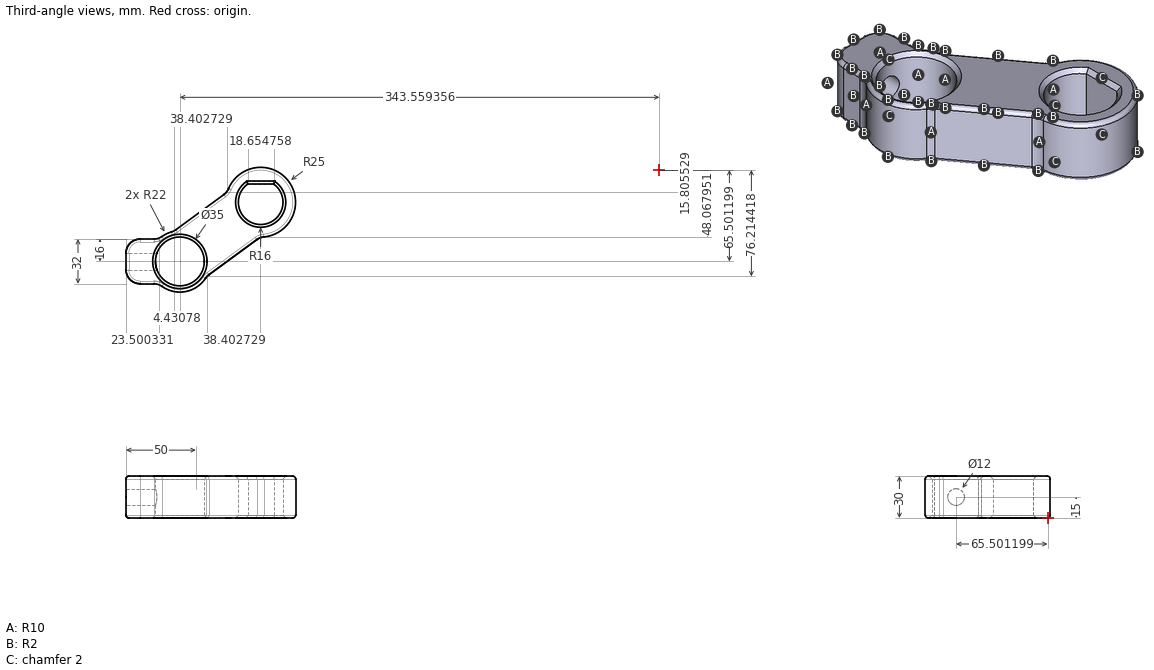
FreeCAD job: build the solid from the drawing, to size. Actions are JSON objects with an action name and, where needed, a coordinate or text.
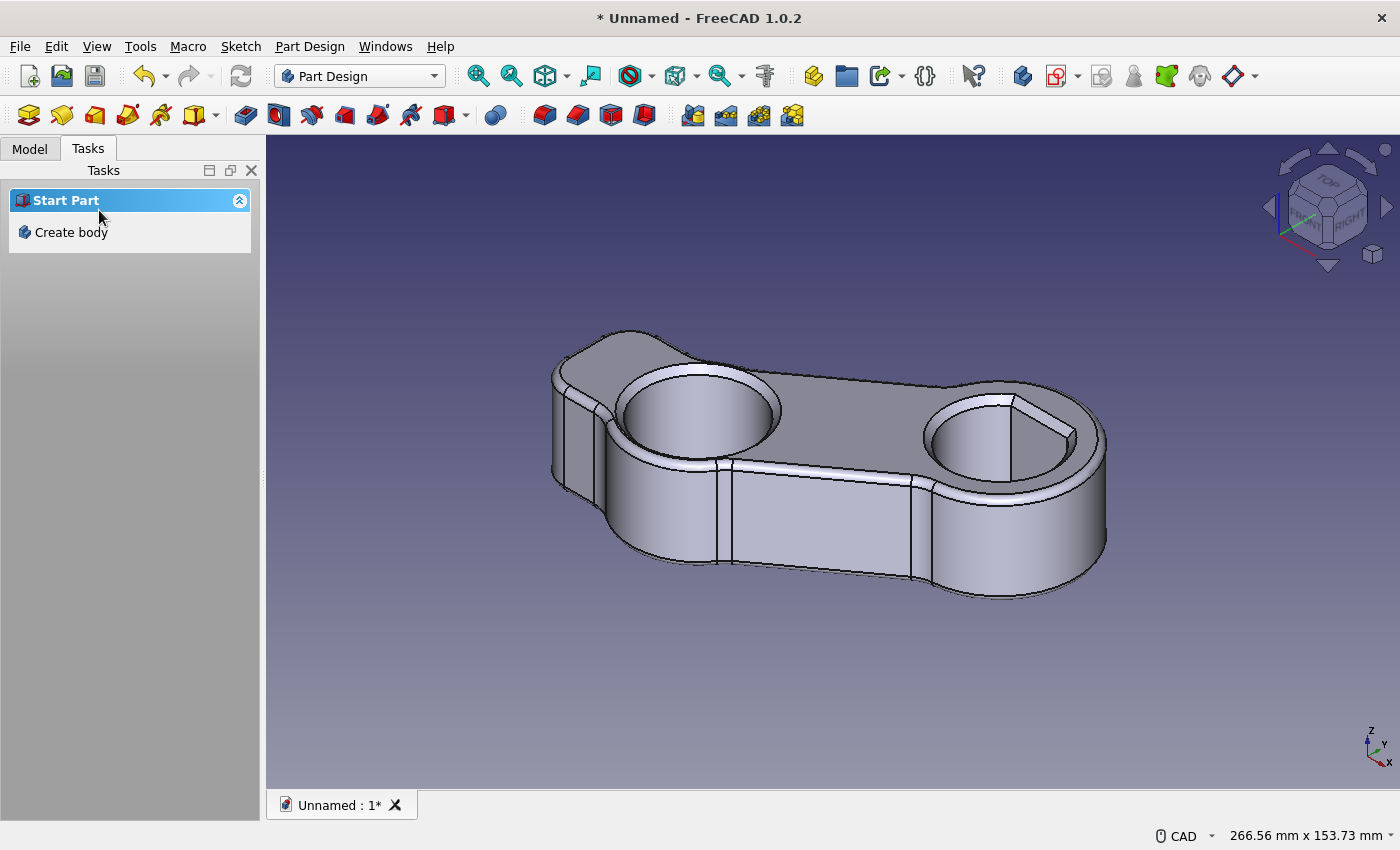
{"action": "key", "text": "6"}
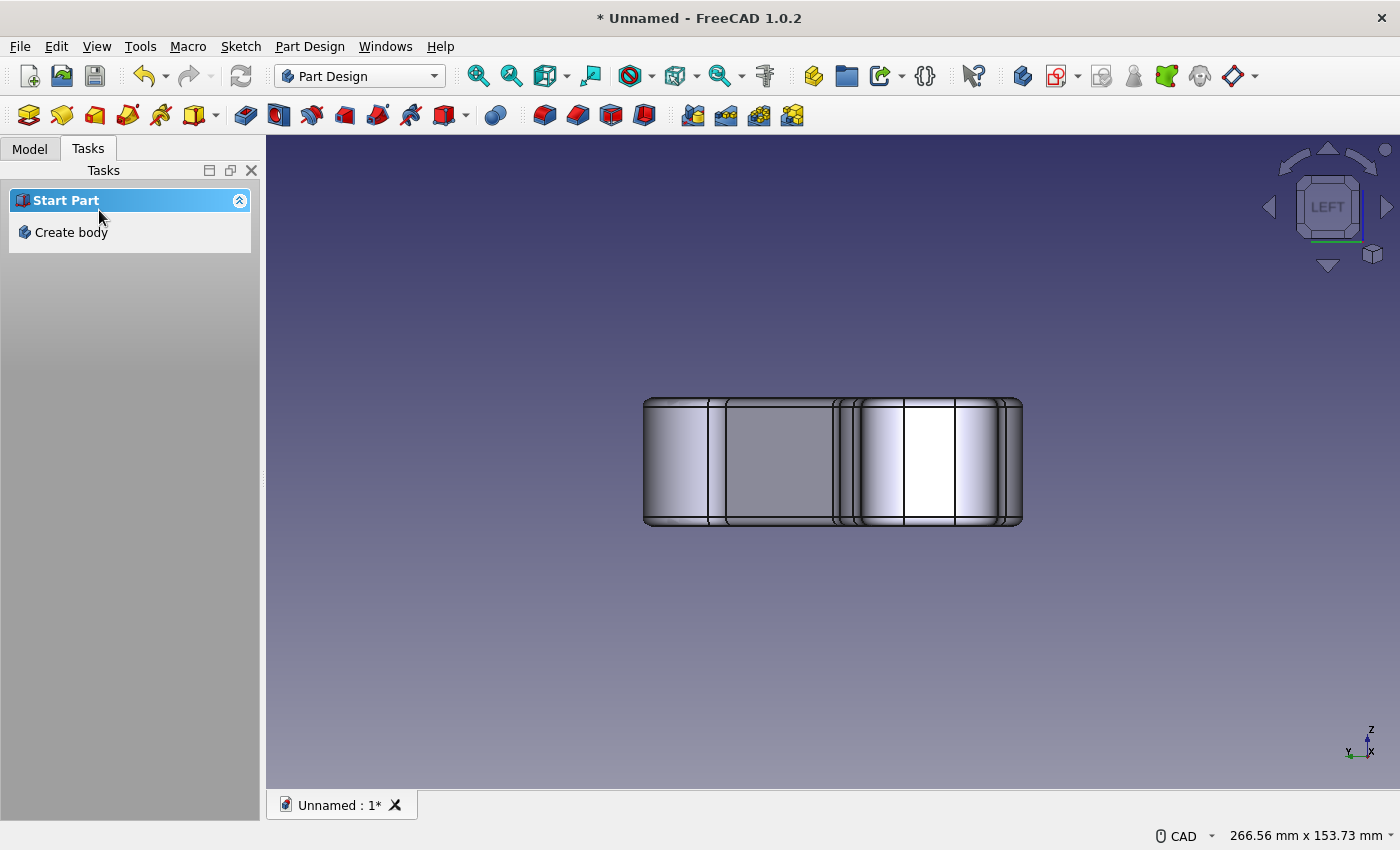
{"action": "key", "text": "v f"}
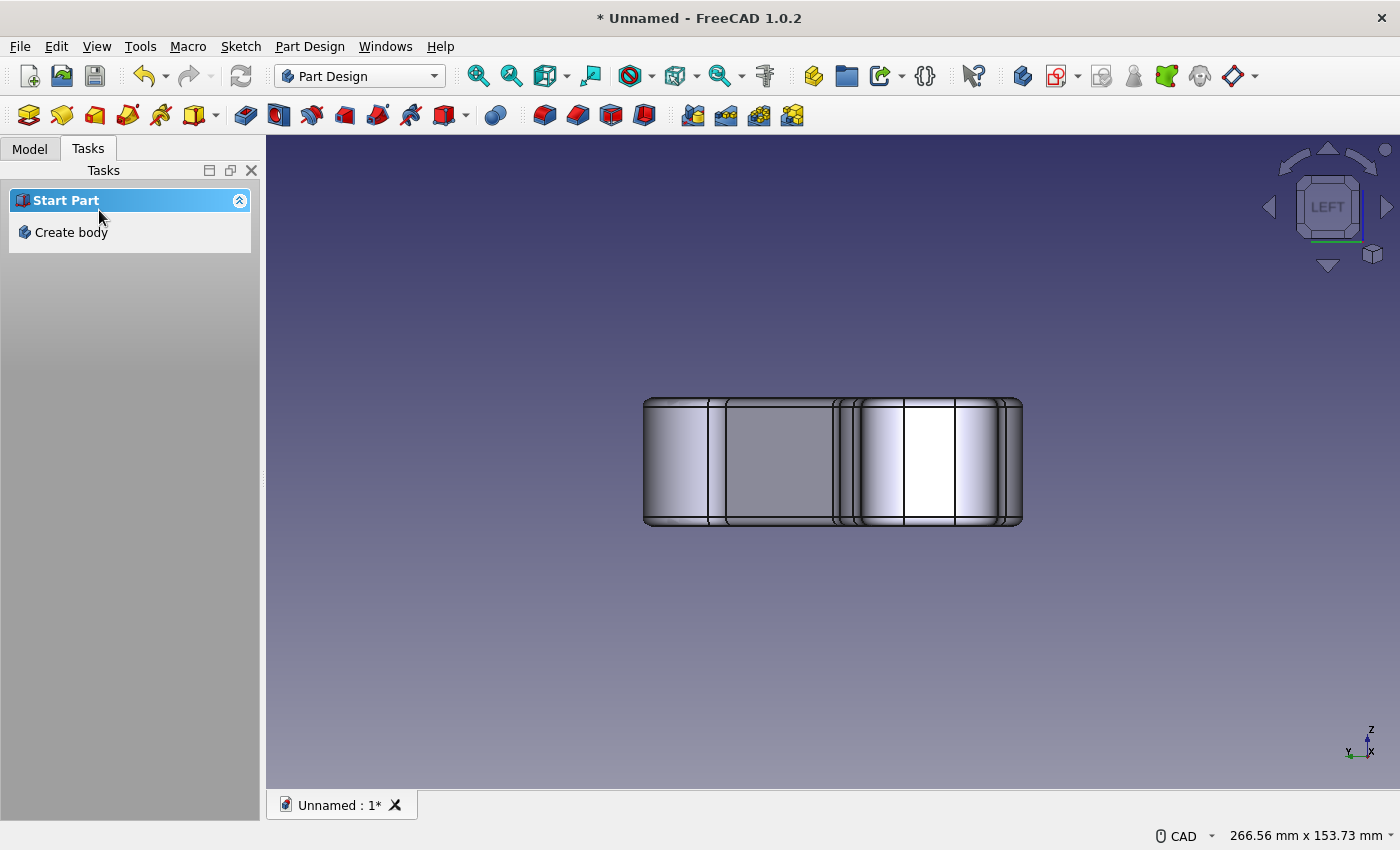
{"action": "left_click", "coordinate": [930, 445]}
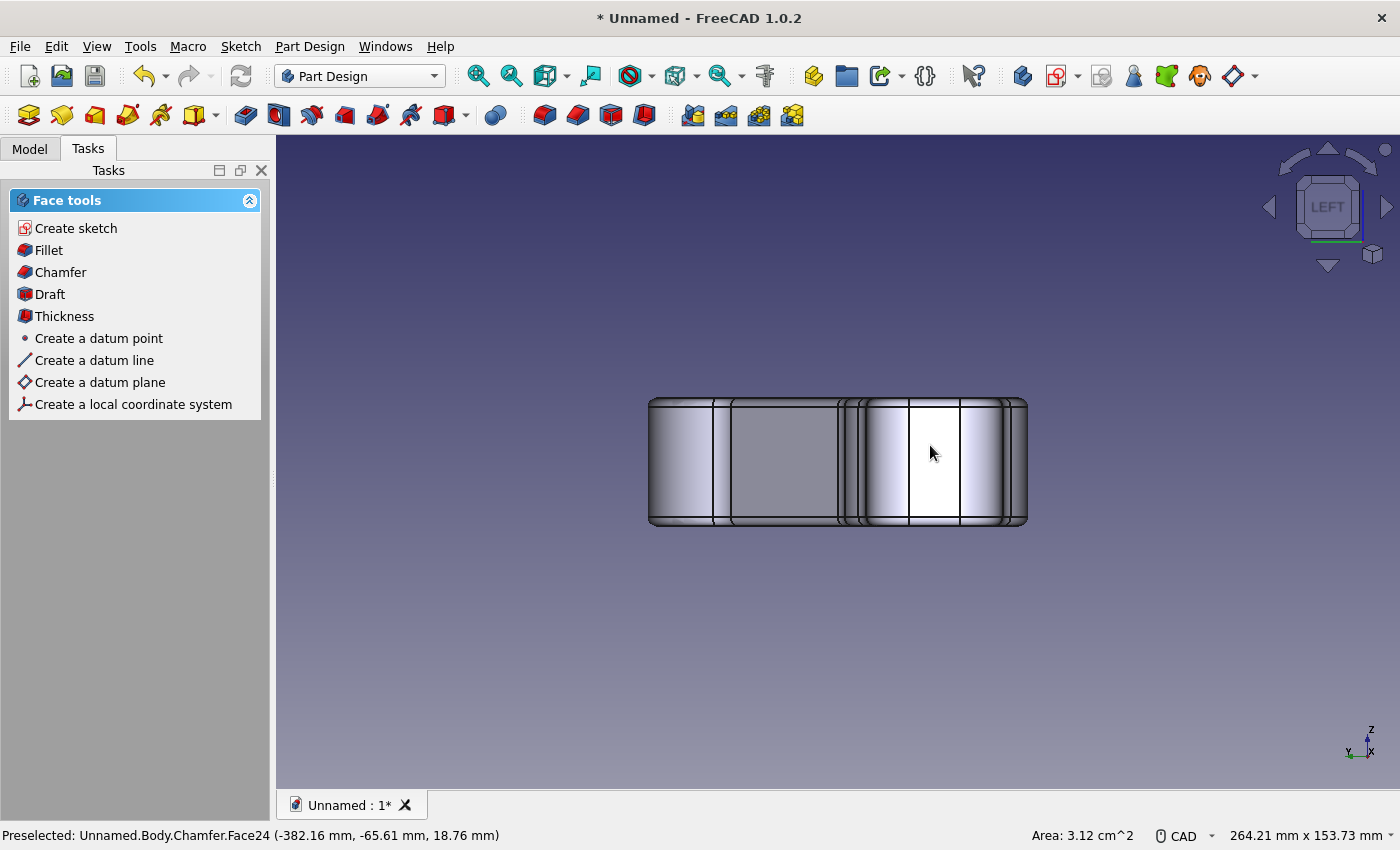
{"action": "left_click", "coordinate": [1056, 76]}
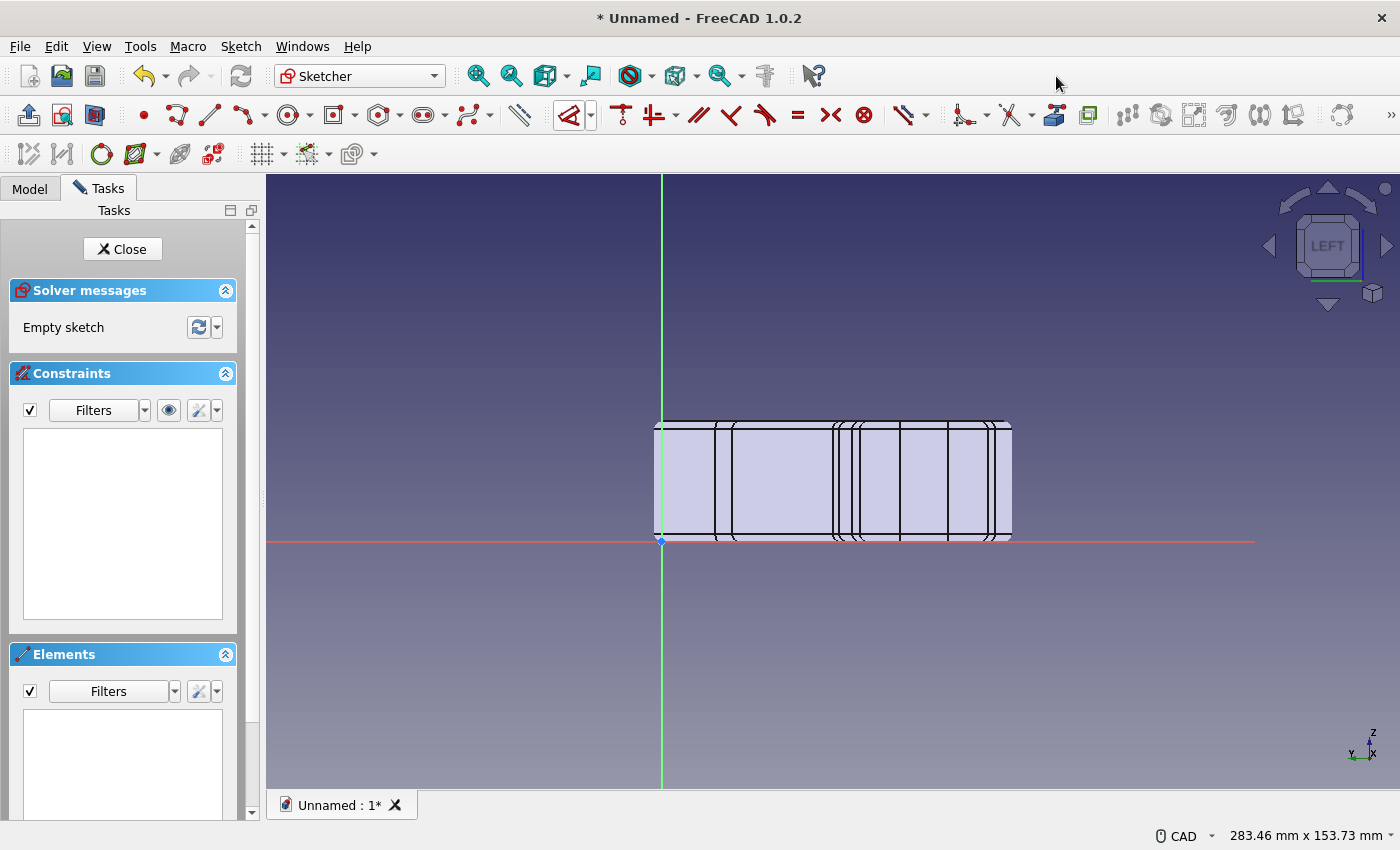
{"action": "scroll", "coordinate": [944, 482], "scroll_direction": "up", "scroll_amount": 11}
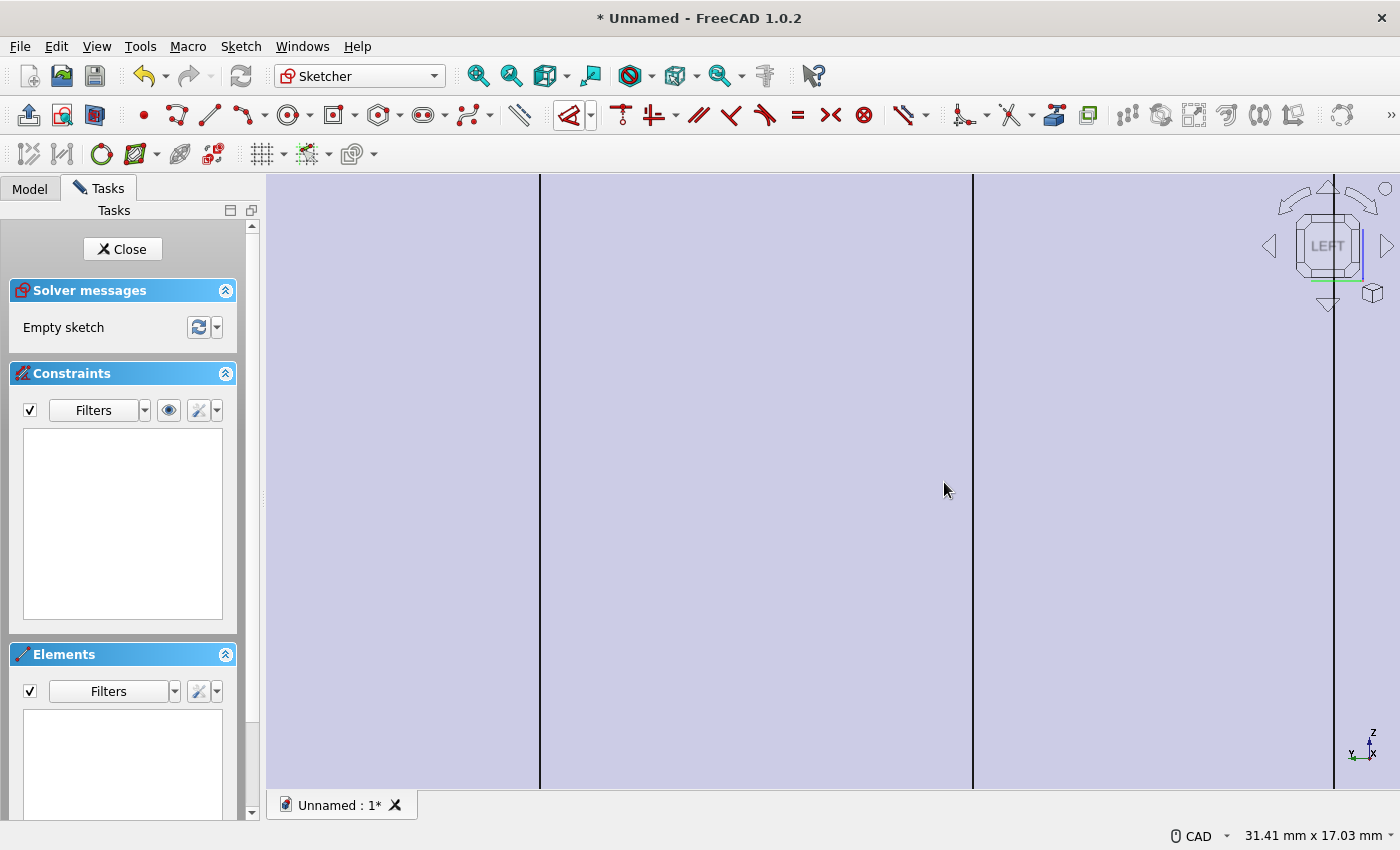
{"action": "left_click", "coordinate": [288, 116]}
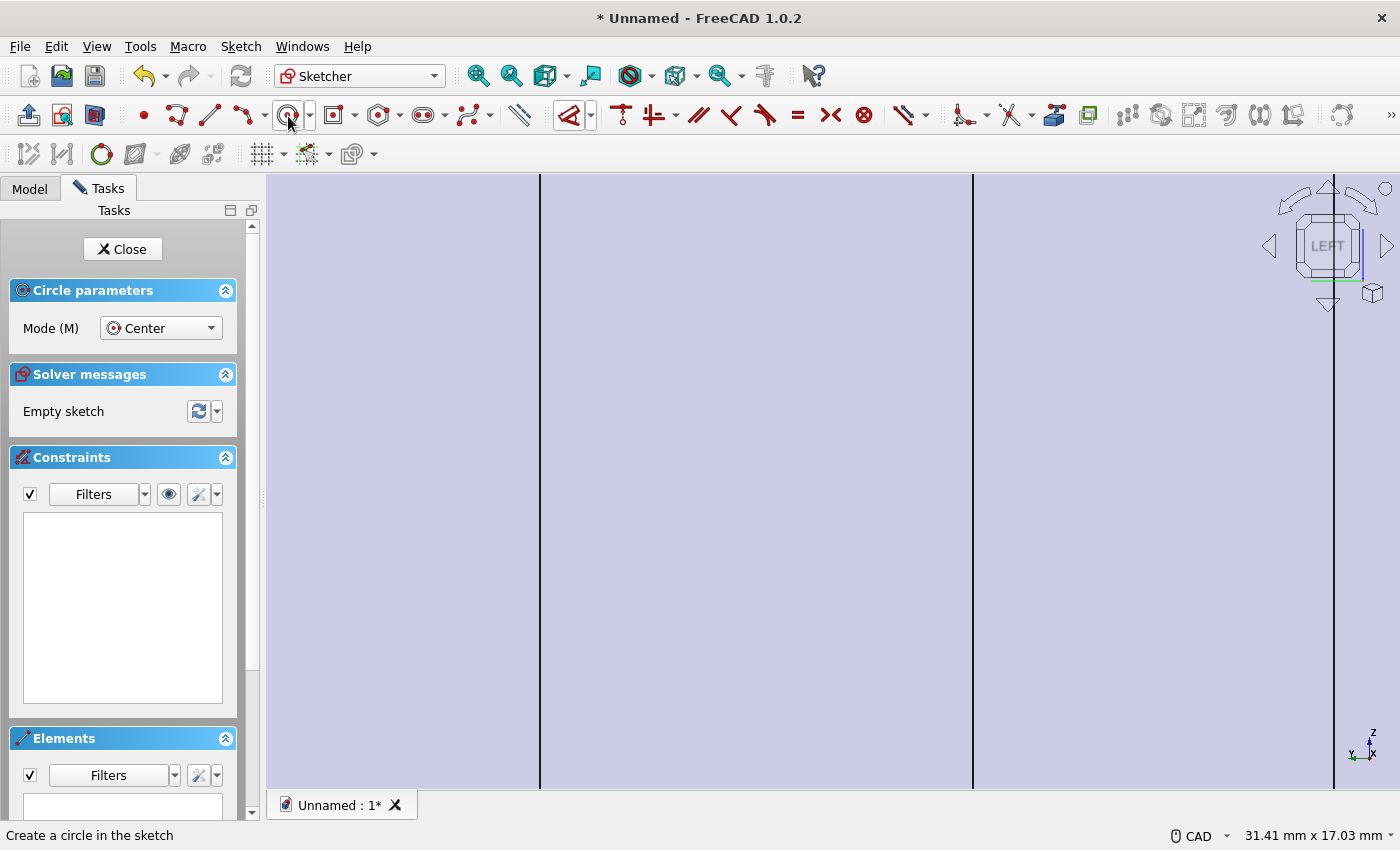
{"action": "left_click", "coordinate": [757, 473]}
{"action": "left_click", "coordinate": [910, 320]}
{"action": "key", "text": "Escape"}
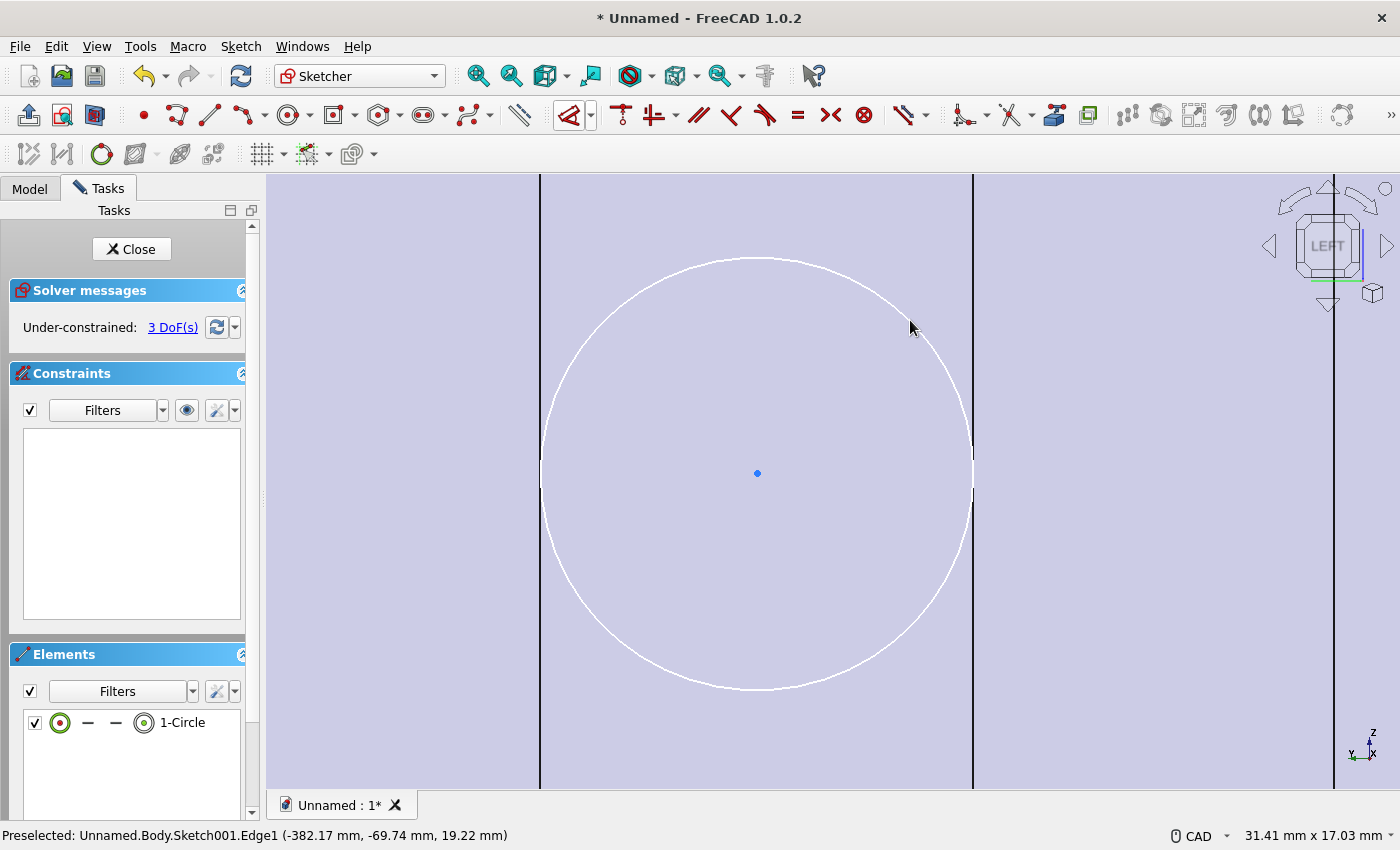
{"action": "left_click", "coordinate": [910, 321]}